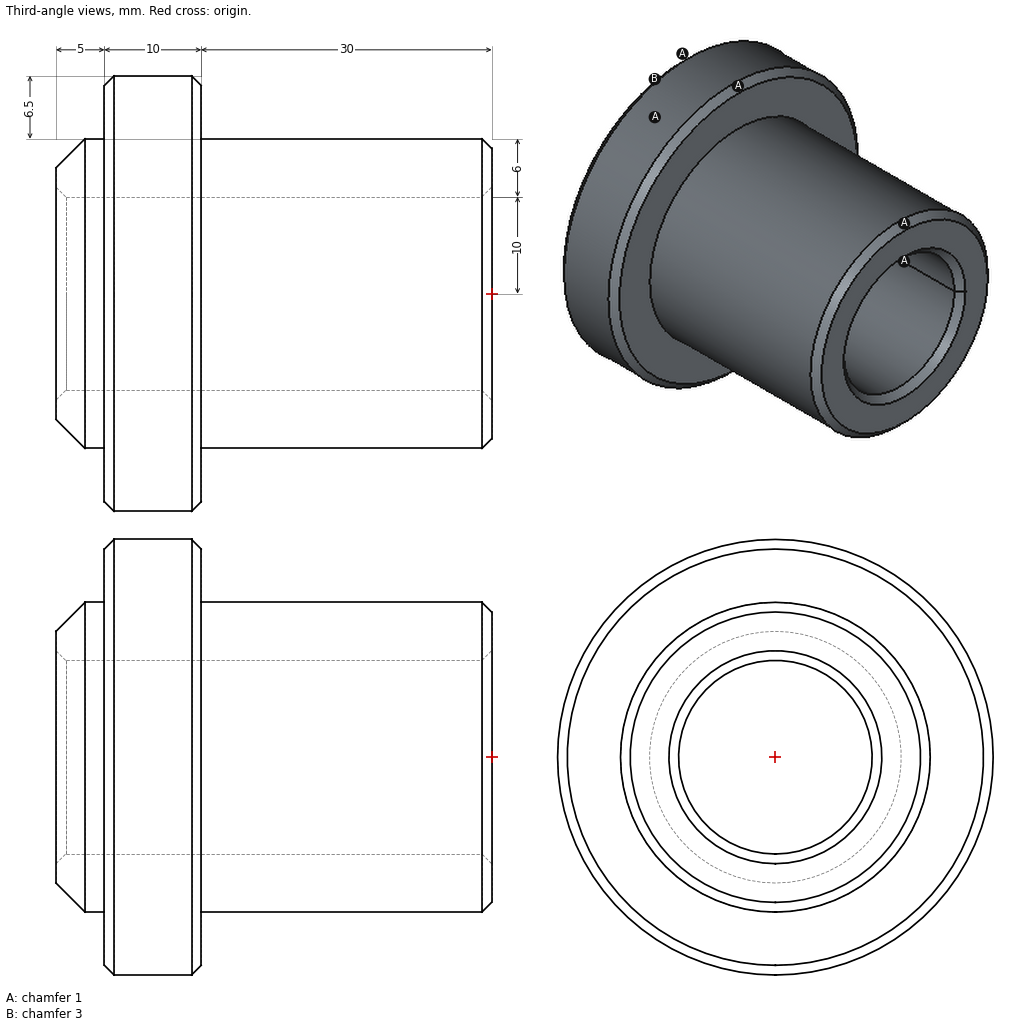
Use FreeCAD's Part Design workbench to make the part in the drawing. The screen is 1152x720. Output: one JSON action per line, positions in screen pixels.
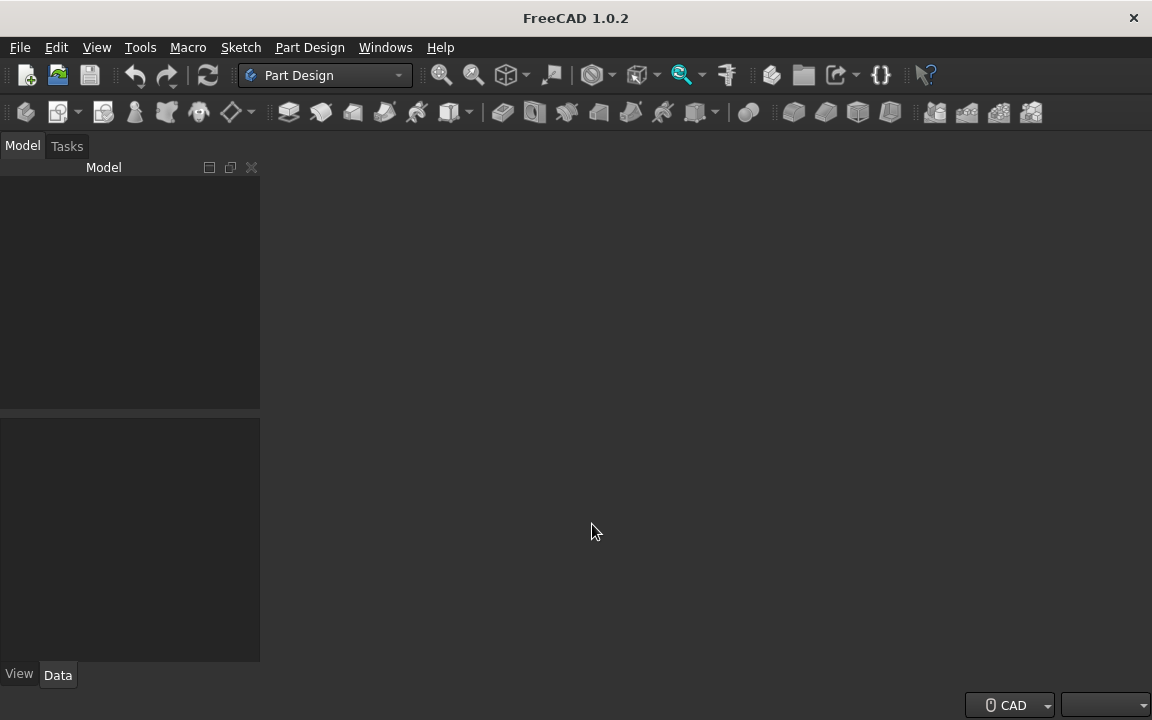
{"action": "left_click", "coordinate": [26, 76]}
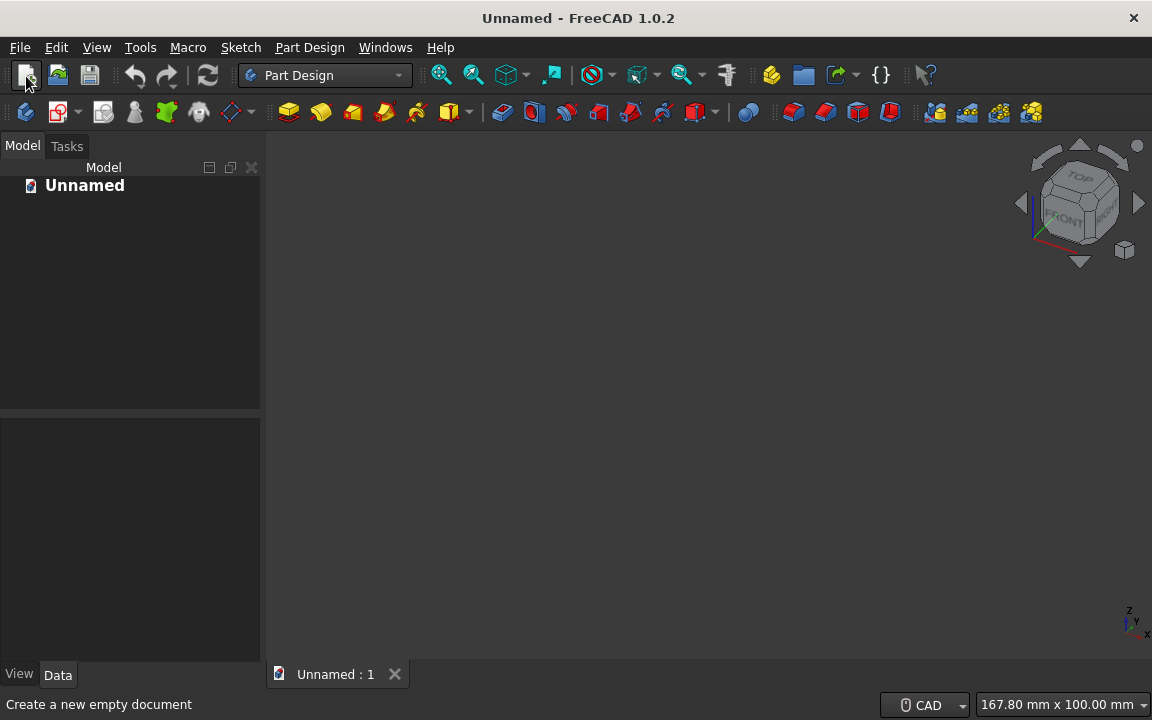
{"action": "left_click", "coordinate": [58, 112]}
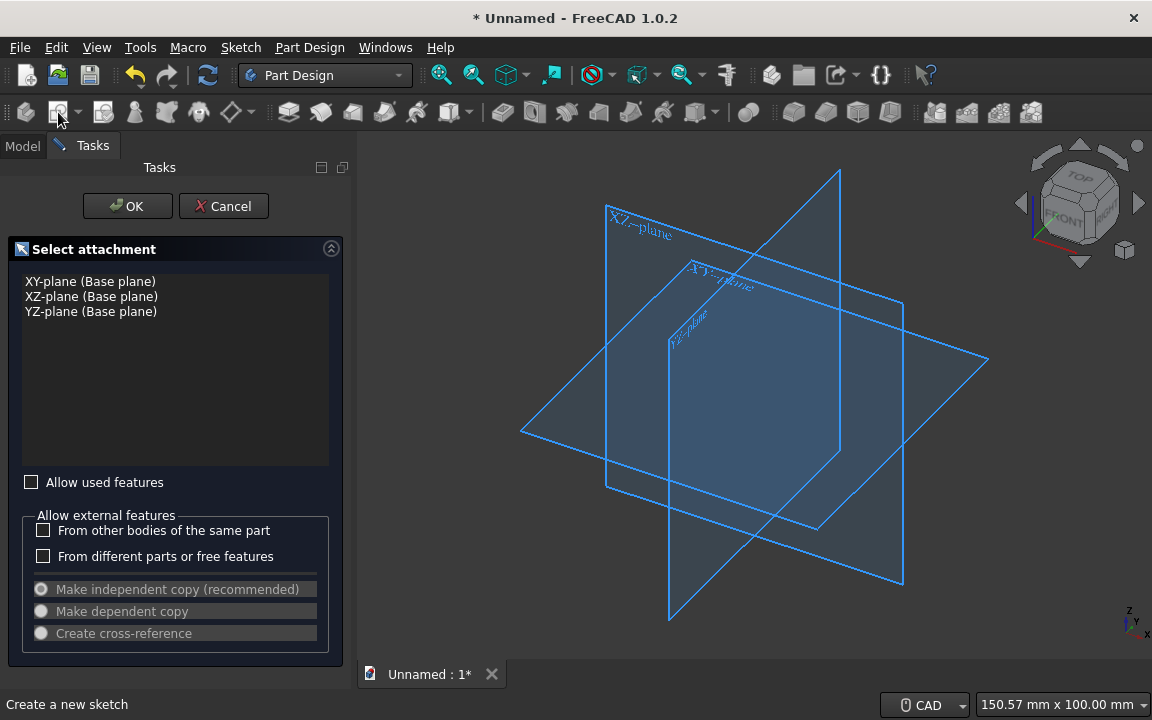
{"action": "left_click", "coordinate": [82, 282]}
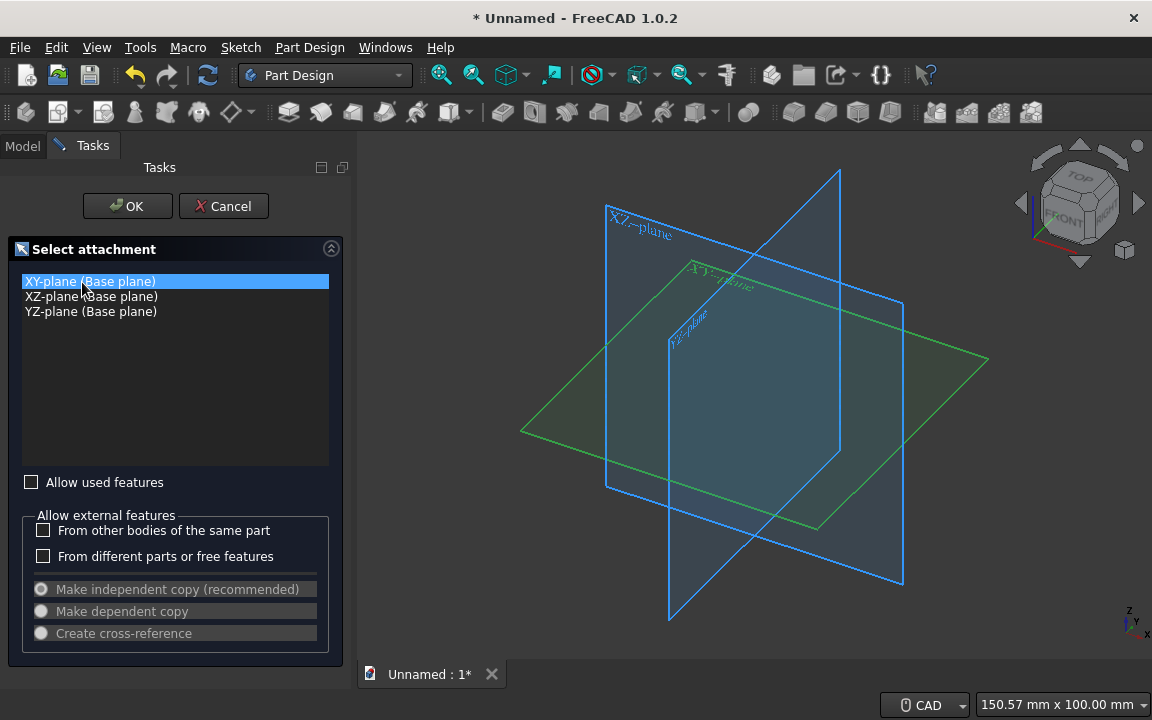
{"action": "left_click", "coordinate": [128, 206]}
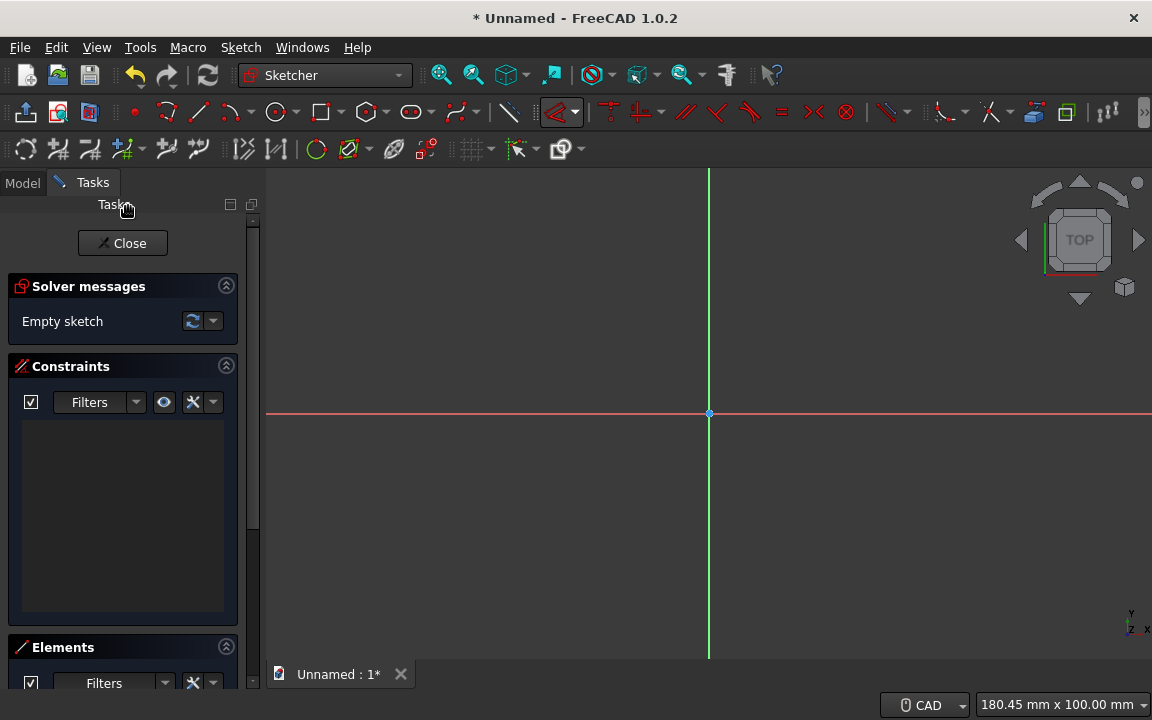
{"action": "scroll", "coordinate": [564, 313], "scroll_direction": "up", "scroll_amount": 4}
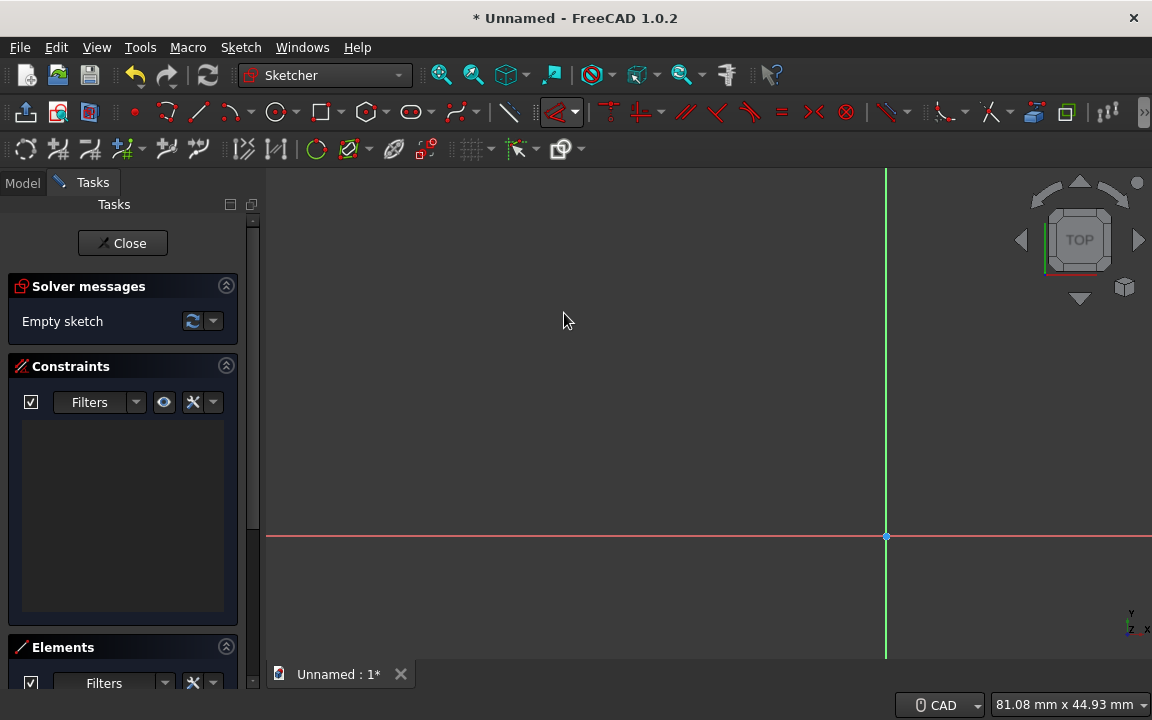
{"action": "left_click", "coordinate": [168, 112]}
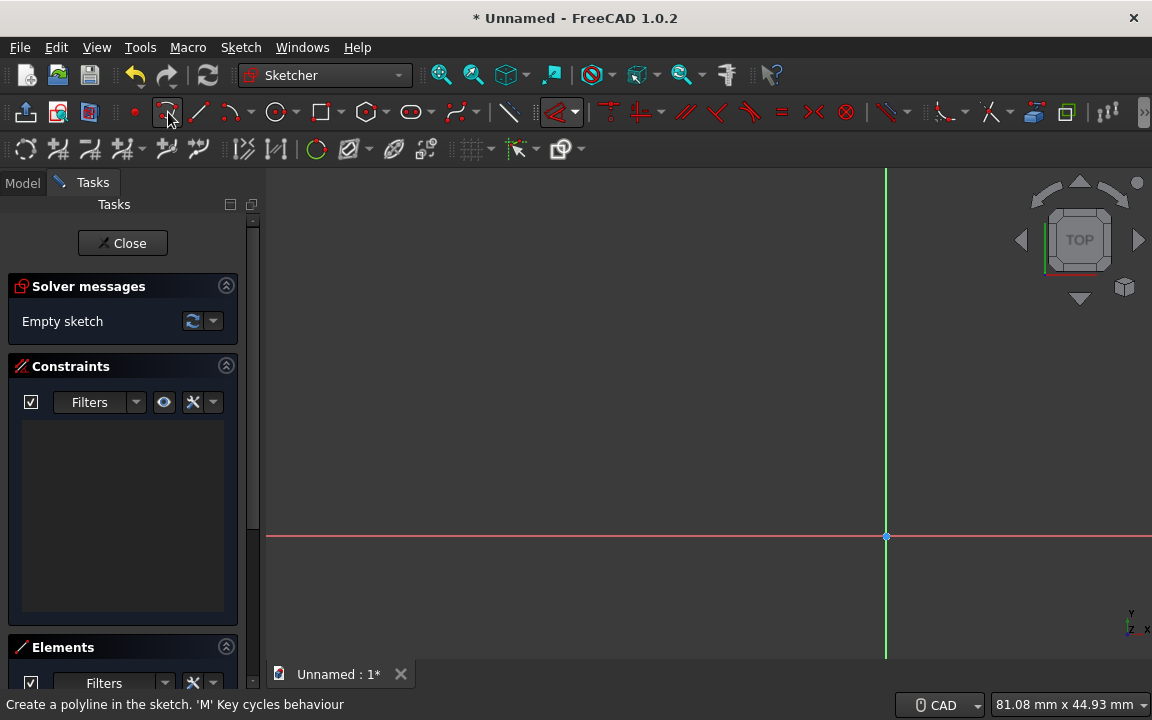
{"action": "left_click", "coordinate": [886, 427]}
{"action": "left_click", "coordinate": [877, 361]}
{"action": "left_click", "coordinate": [558, 361]}
{"action": "left_click", "coordinate": [558, 290]}
{"action": "left_click", "coordinate": [449, 290]}
{"action": "left_click", "coordinate": [449, 361]}
{"action": "left_click", "coordinate": [395, 361]}
{"action": "left_click", "coordinate": [395, 427]}
{"action": "left_click", "coordinate": [886, 428]}
{"action": "key", "text": "Escape"}
{"action": "key", "text": "Escape"}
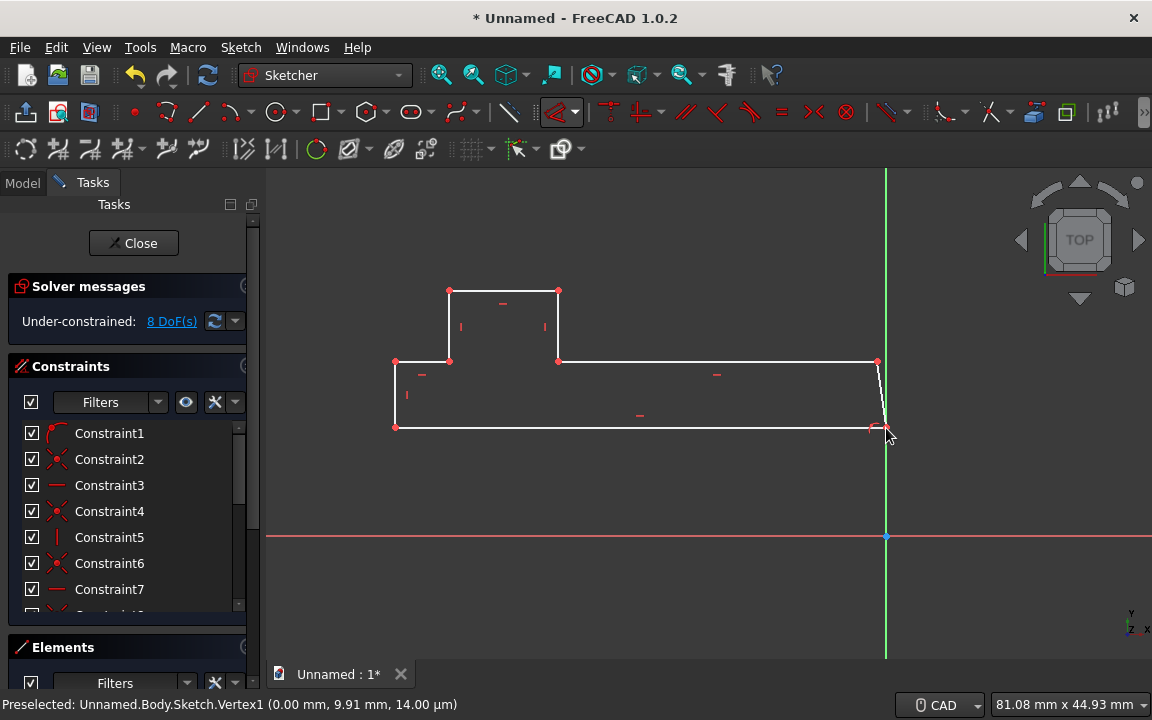
{"action": "left_click", "coordinate": [884, 408]}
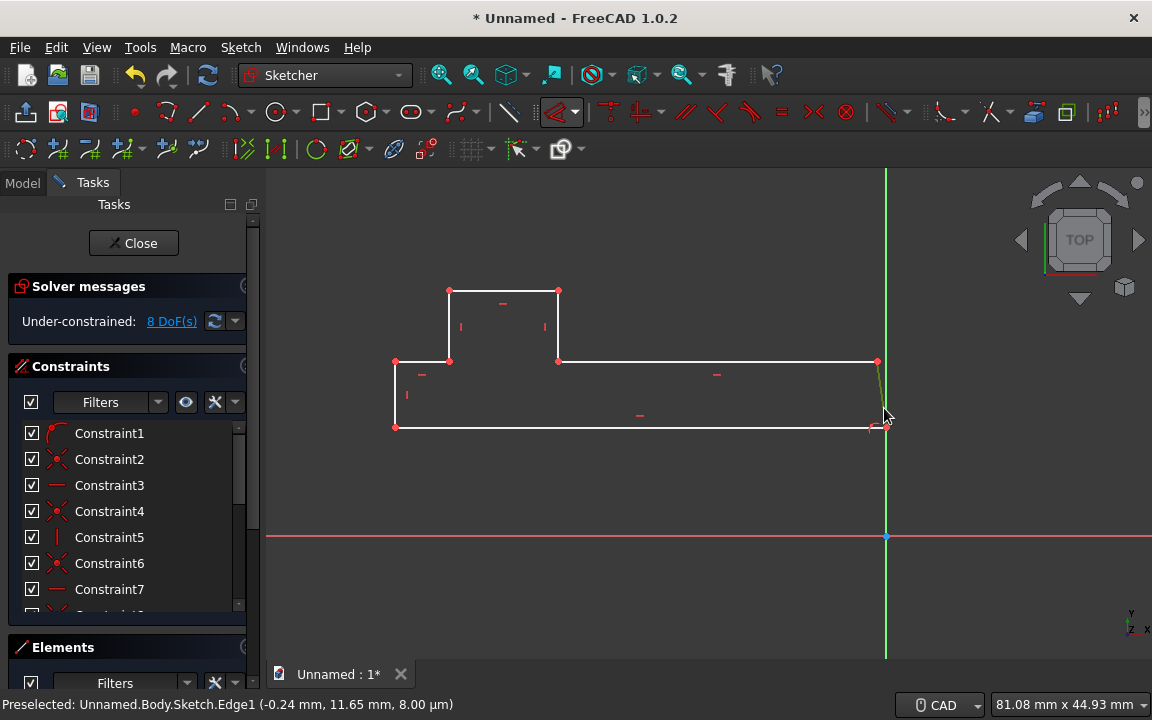
{"action": "left_click", "coordinate": [664, 112]}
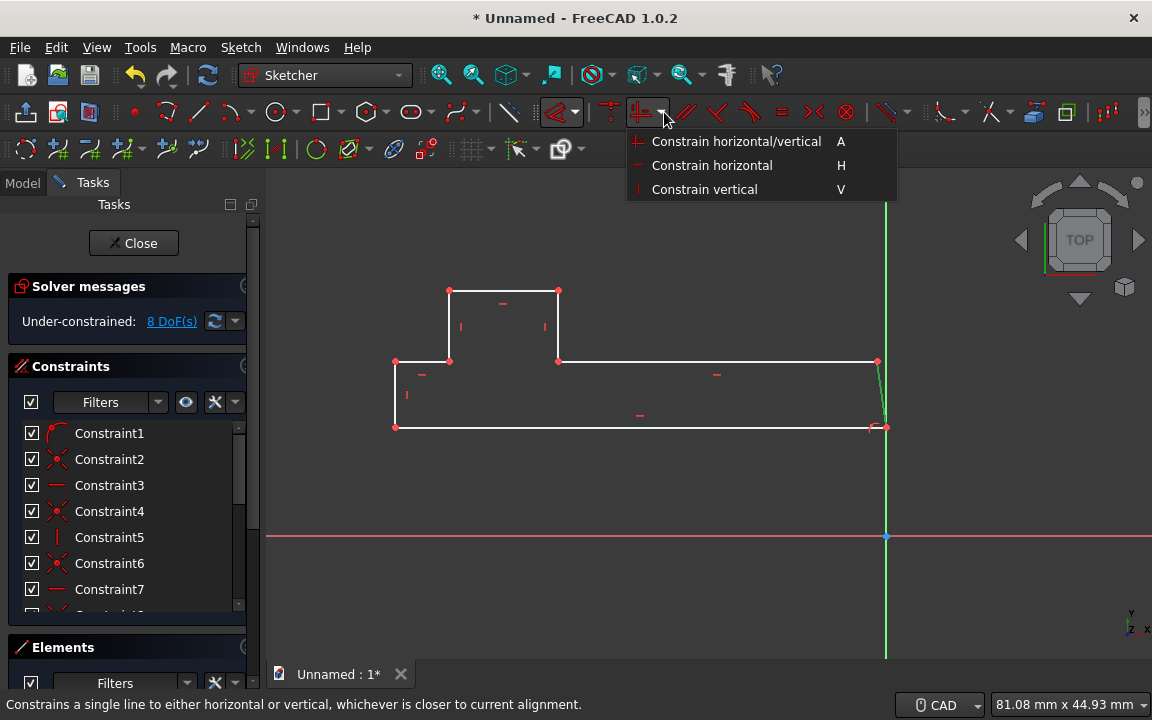
{"action": "left_click", "coordinate": [762, 189]}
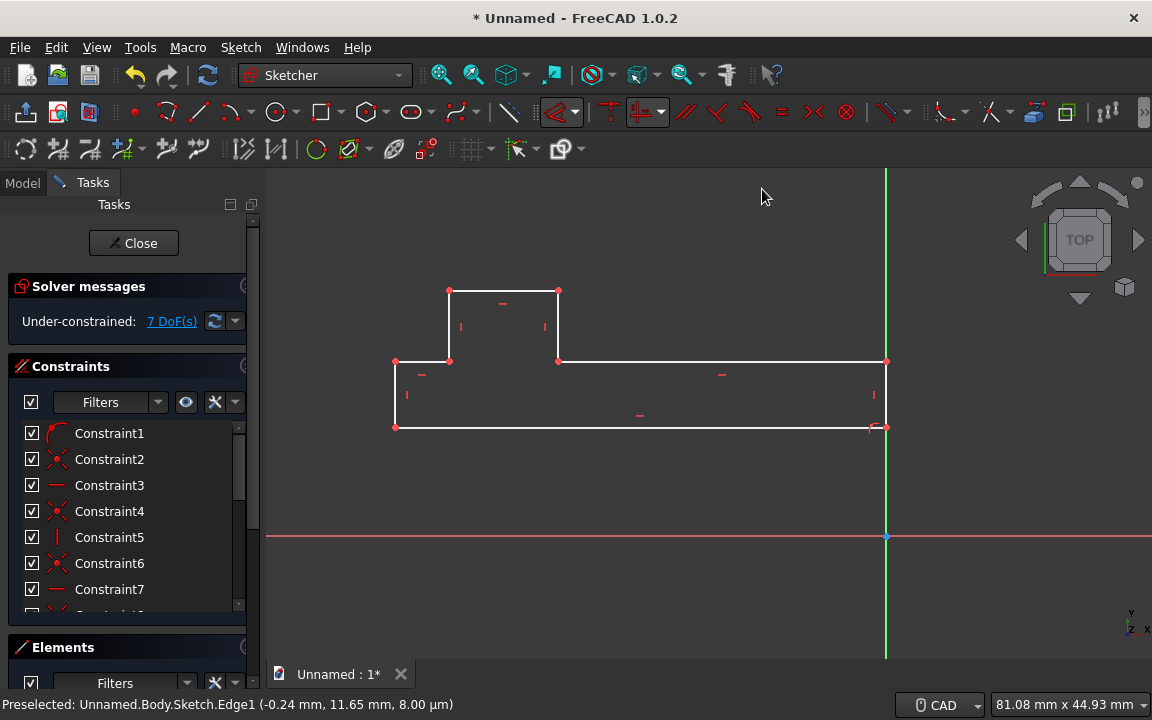
{"action": "left_click", "coordinate": [556, 112]}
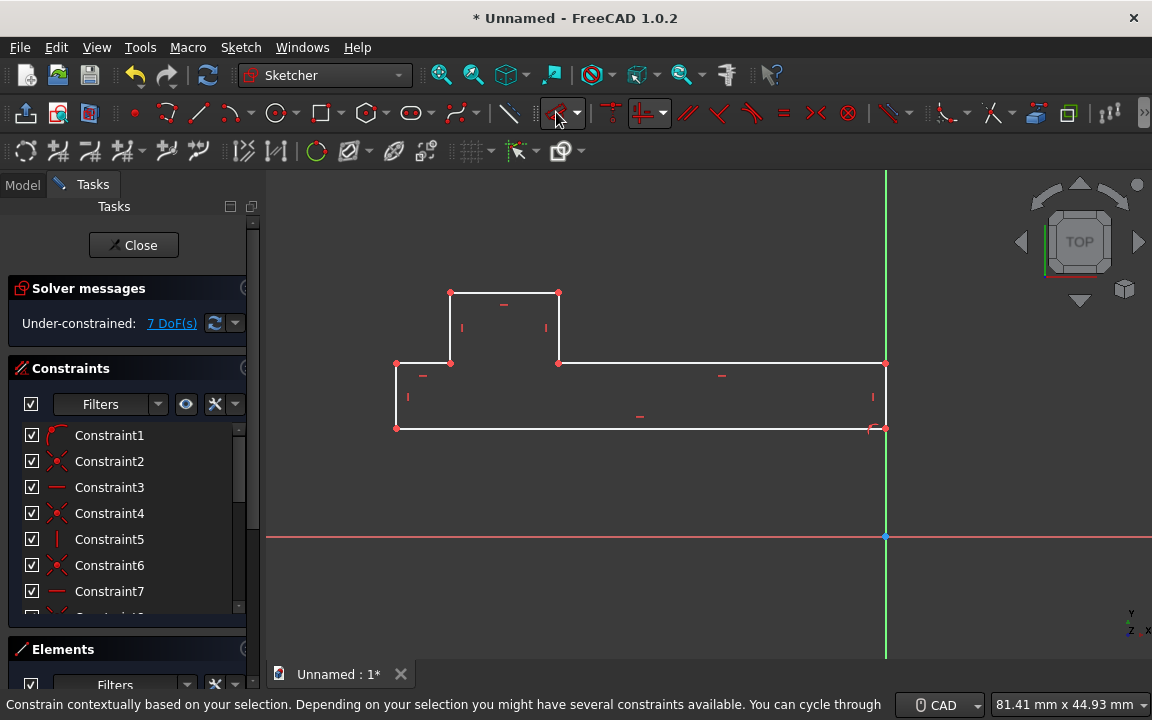
{"action": "left_click", "coordinate": [886, 409]}
{"action": "left_click", "coordinate": [920, 396]}